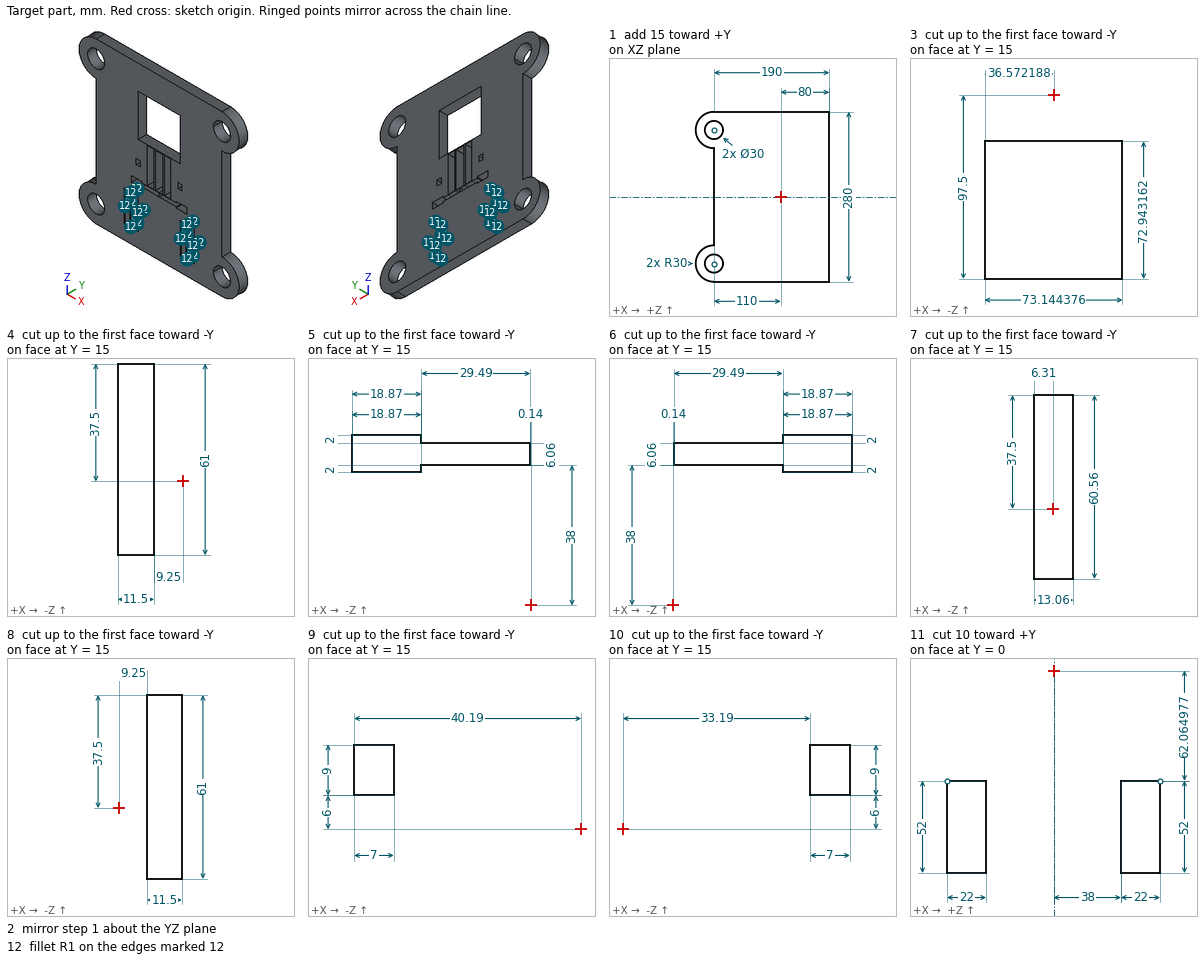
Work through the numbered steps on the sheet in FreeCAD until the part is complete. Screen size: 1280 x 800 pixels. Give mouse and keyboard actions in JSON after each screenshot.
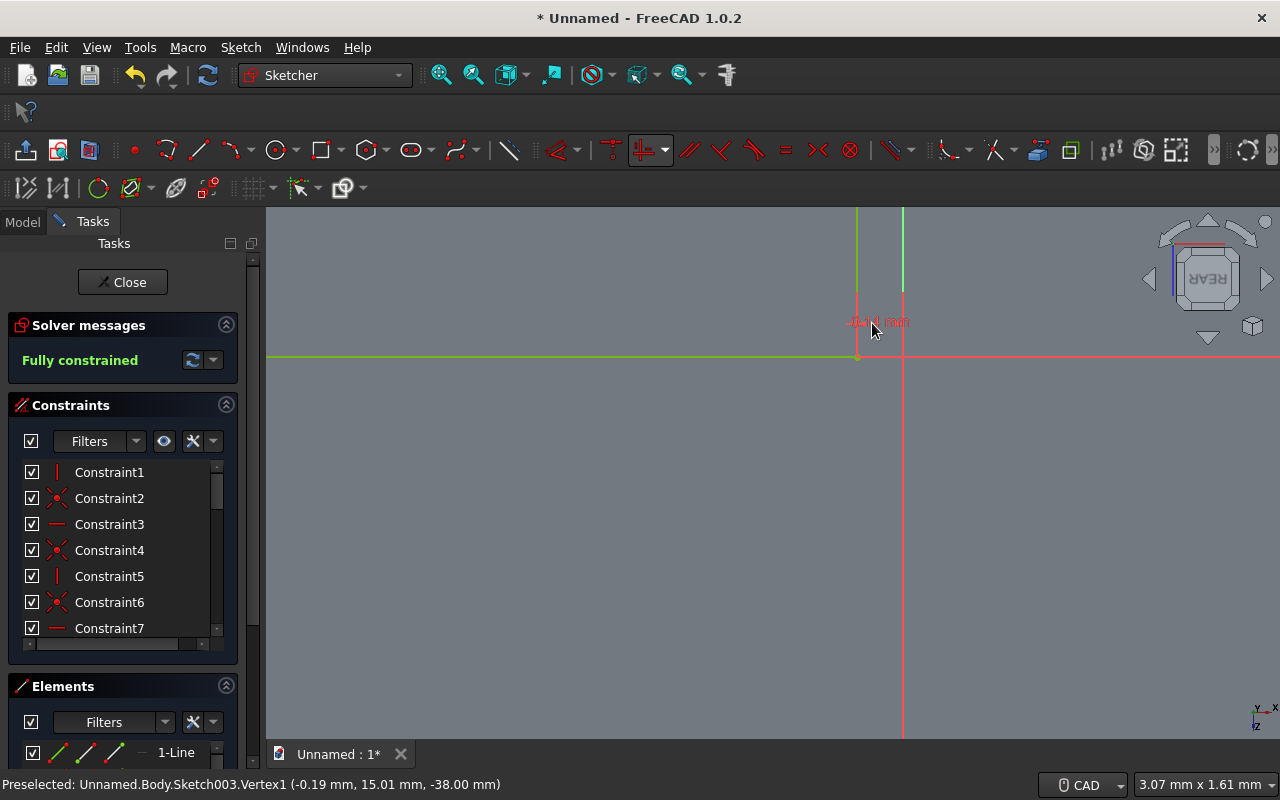
{"action": "left_click", "coordinate": [123, 282]}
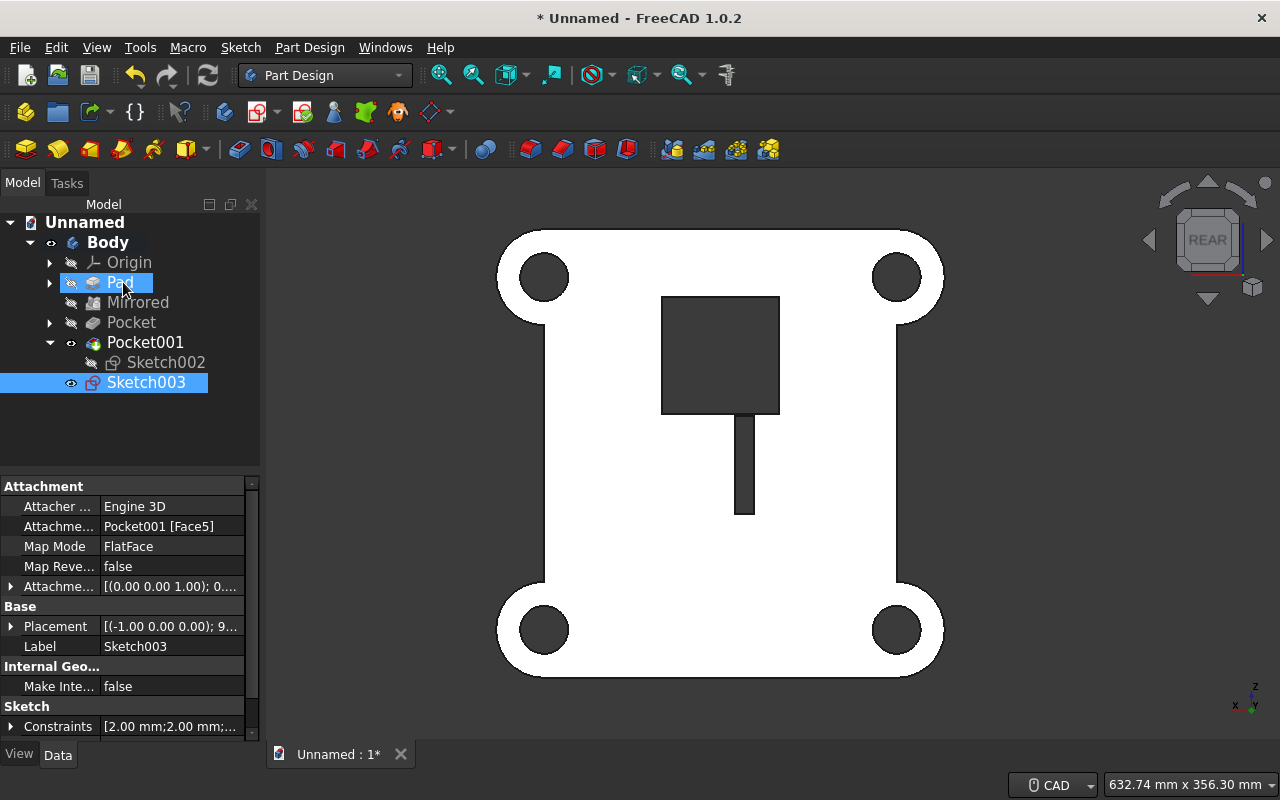
{"action": "left_click", "coordinate": [240, 150]}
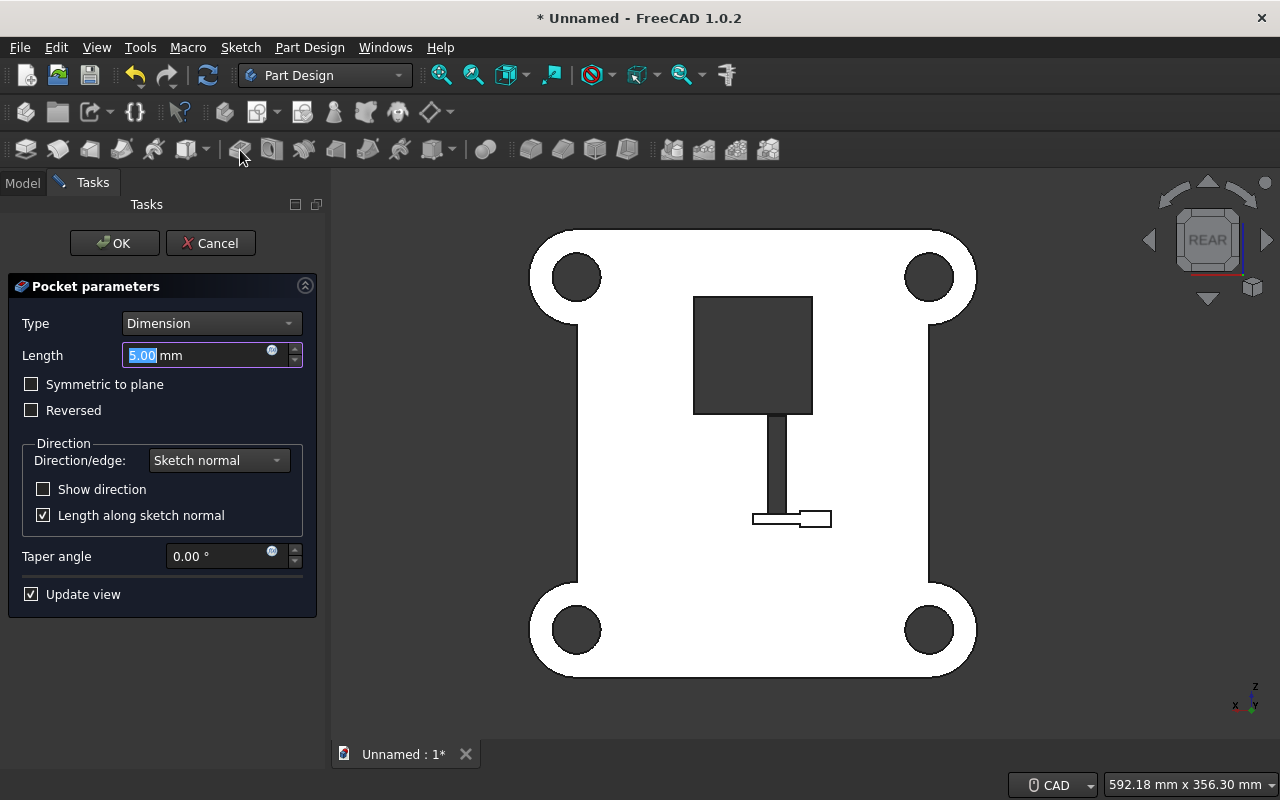
{"action": "left_click", "coordinate": [212, 324]}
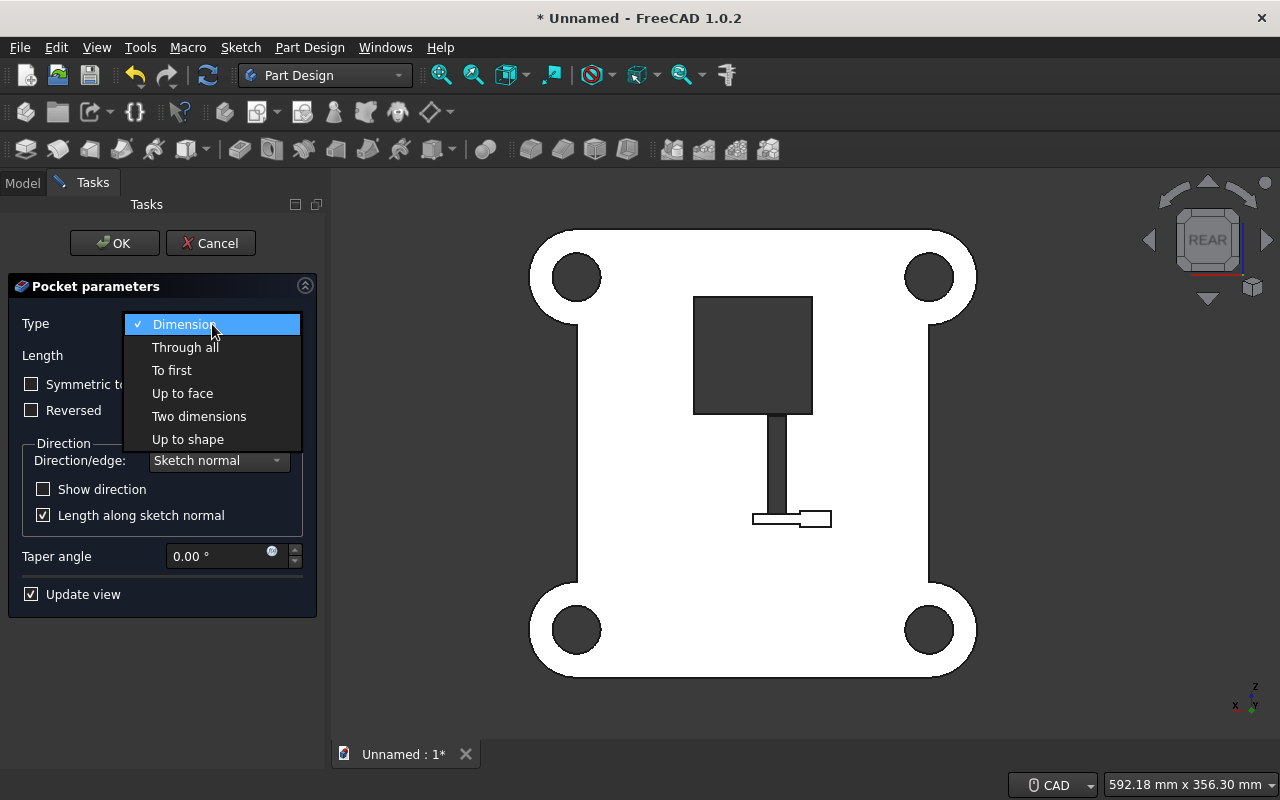
{"action": "left_click", "coordinate": [212, 370]}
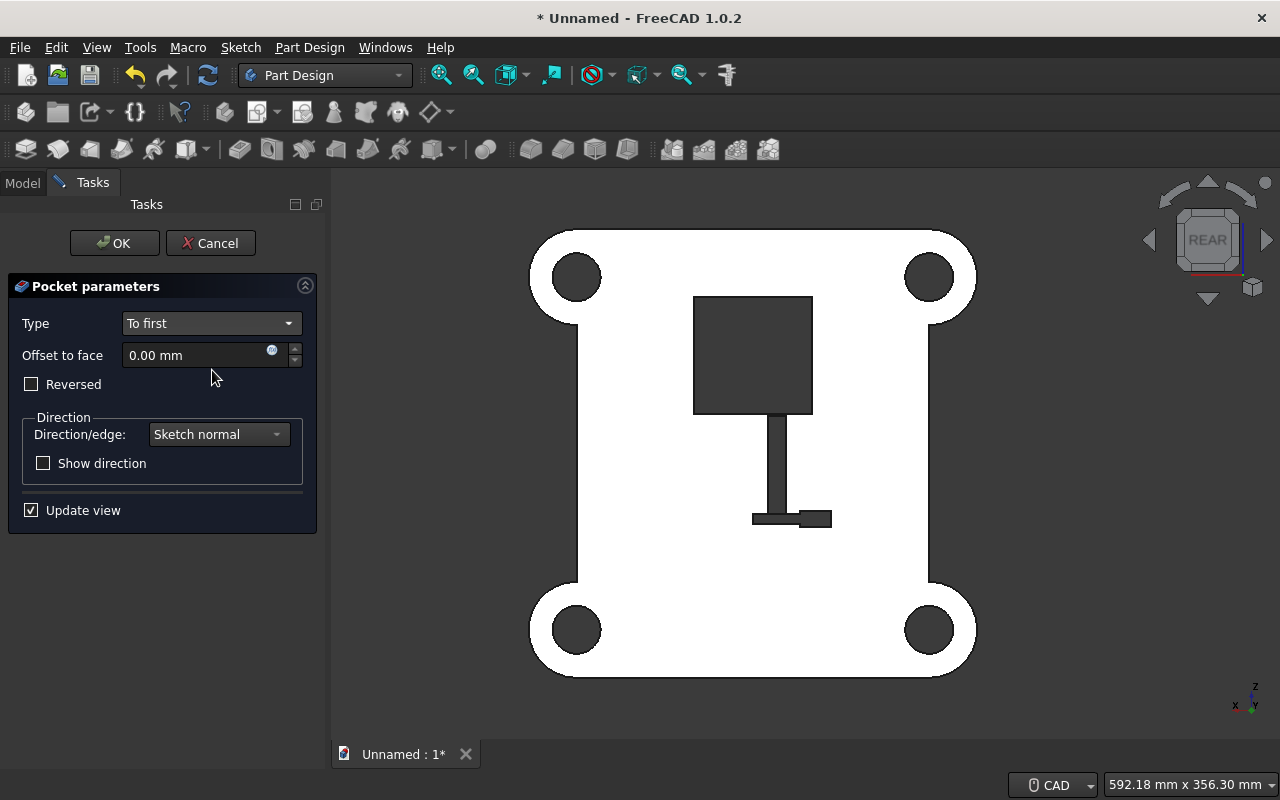
{"action": "left_click", "coordinate": [115, 243]}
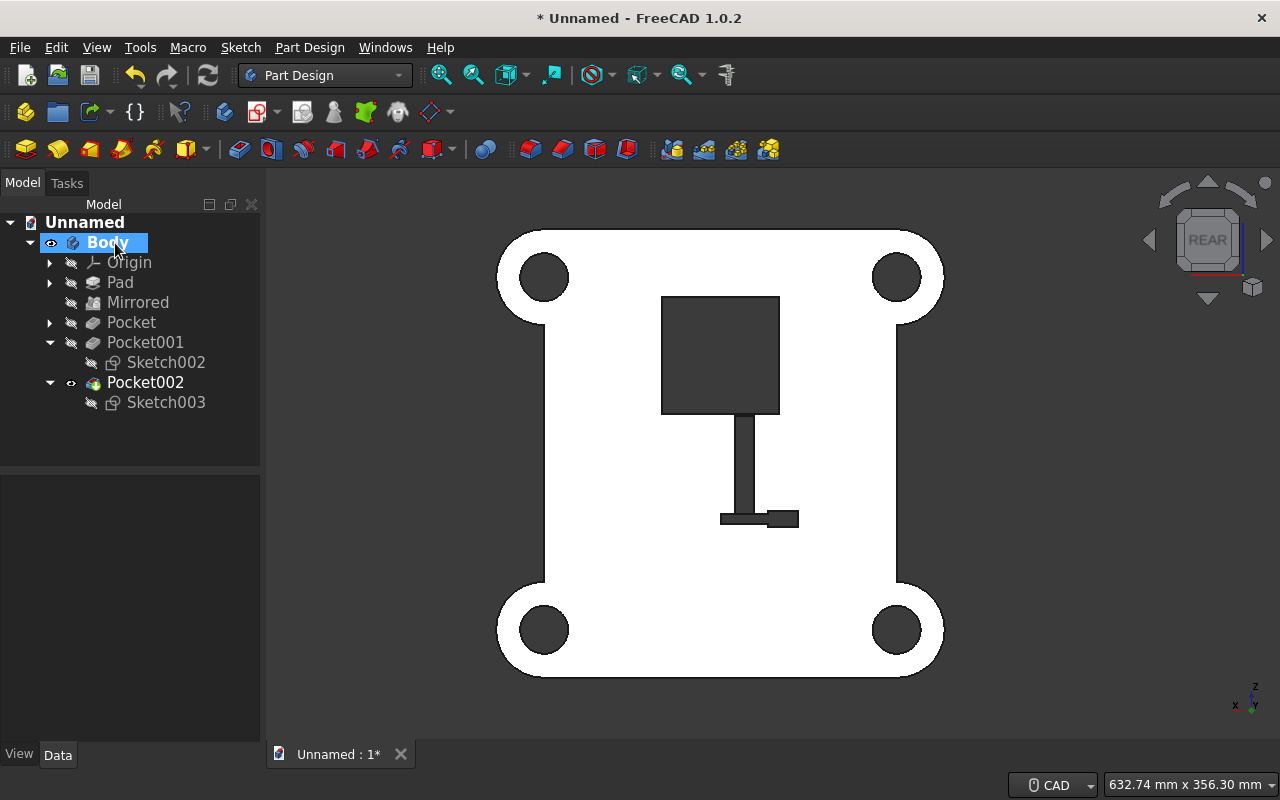
{"action": "left_click", "coordinate": [656, 581]}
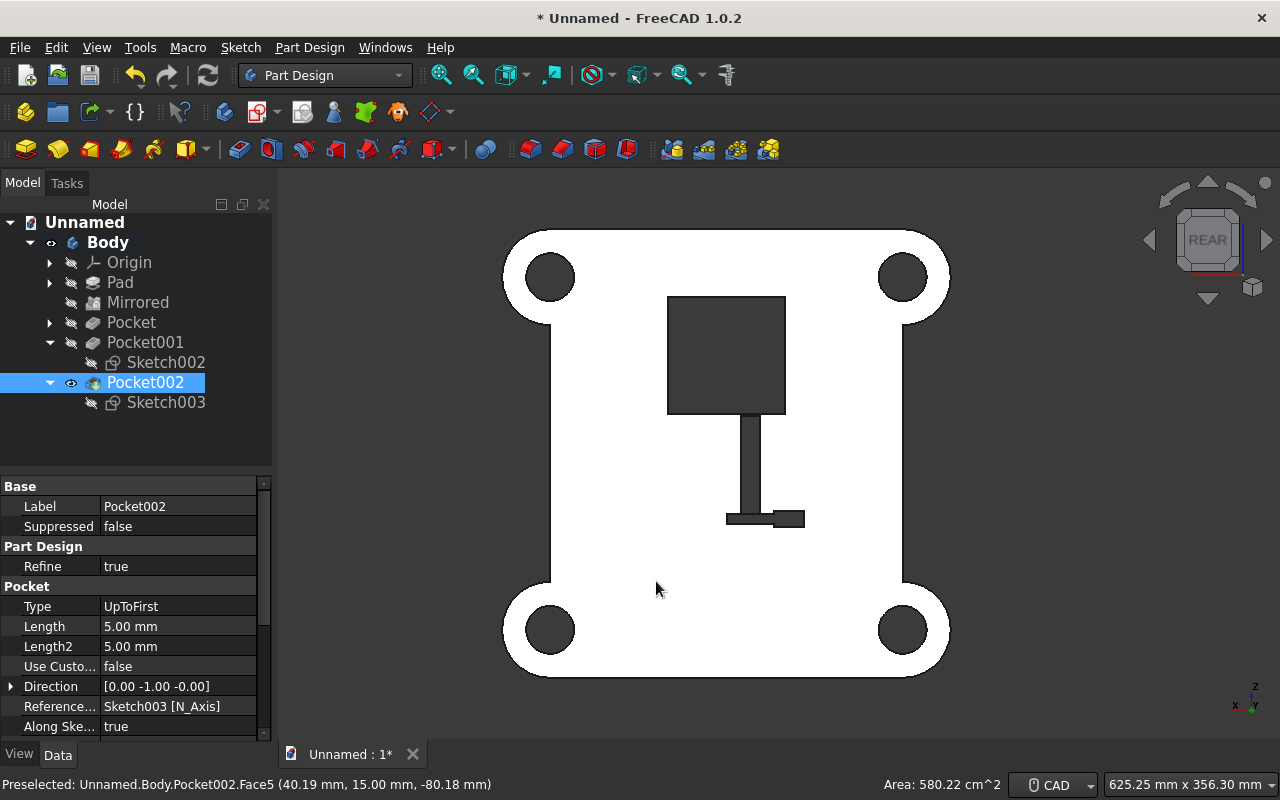
{"action": "left_click", "coordinate": [258, 112]}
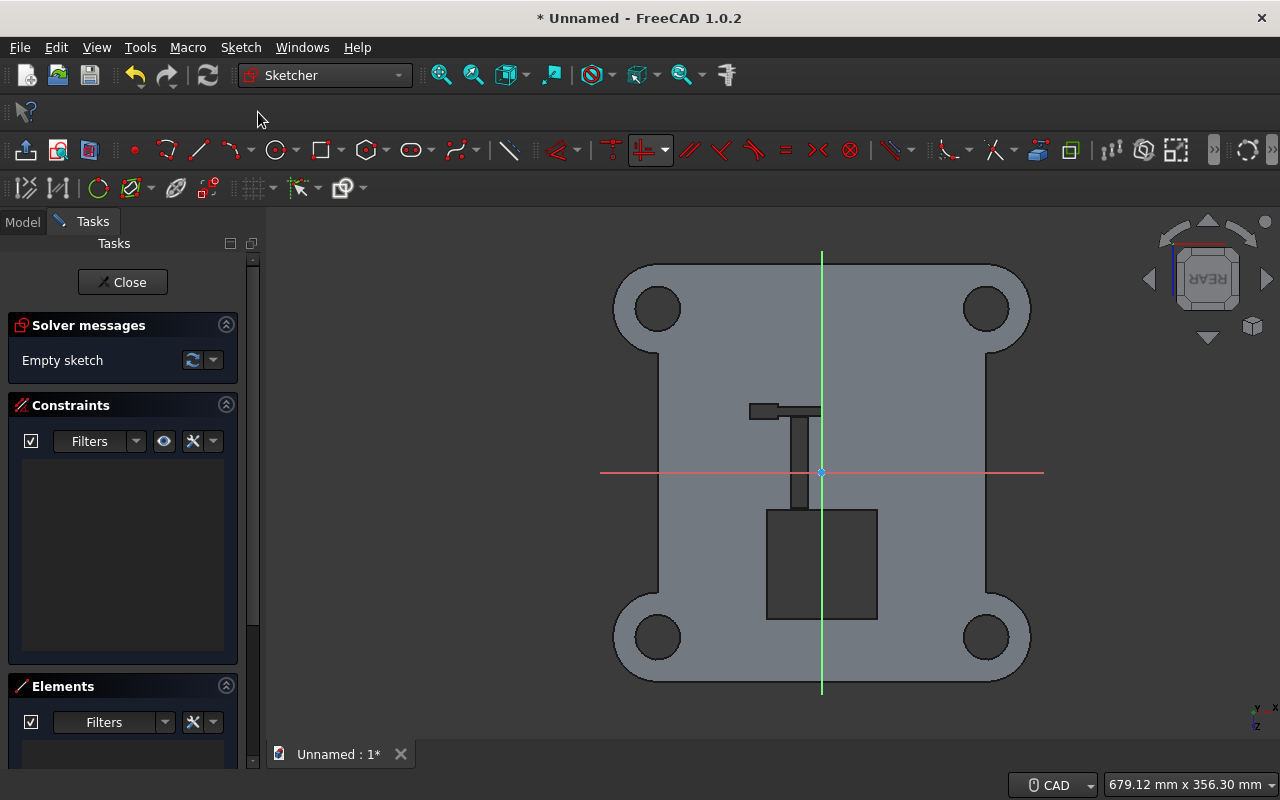
{"action": "scroll", "coordinate": [897, 430], "scroll_direction": "up", "scroll_amount": 8}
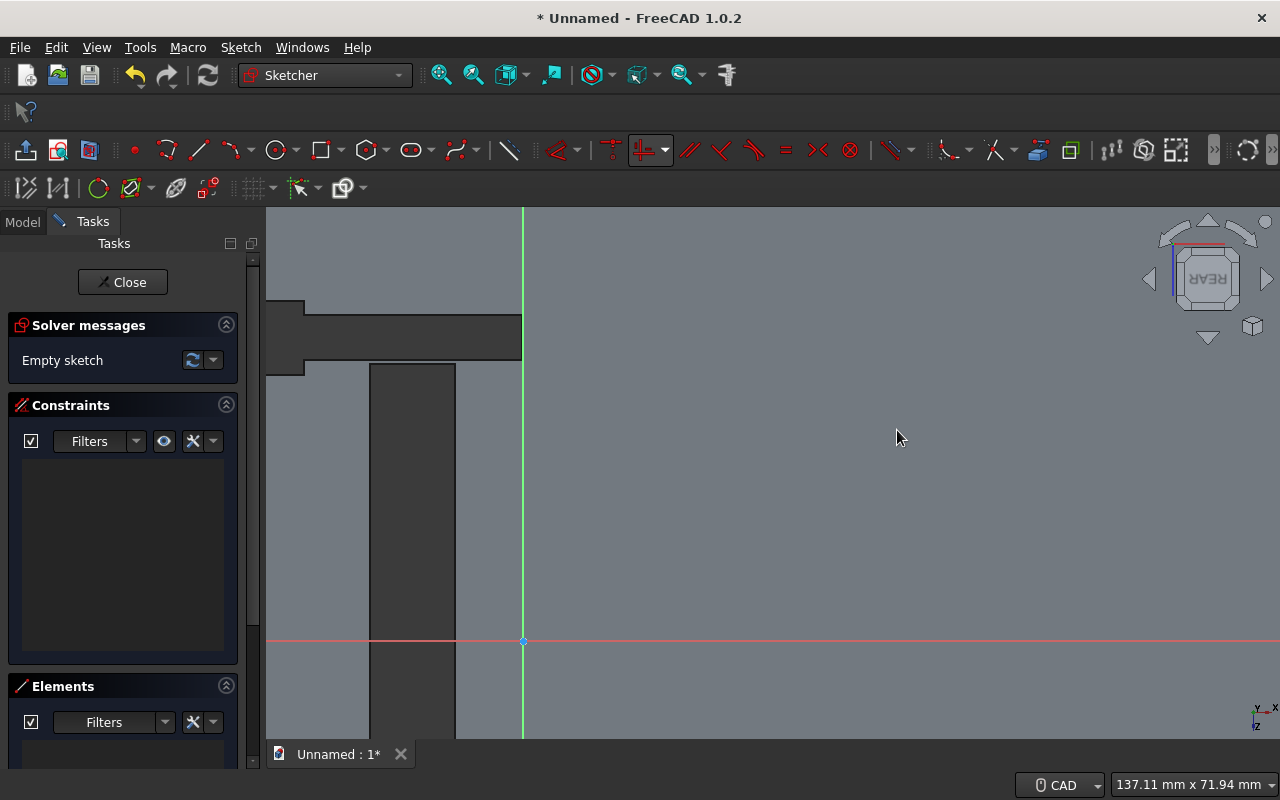
{"action": "left_click", "coordinate": [168, 150]}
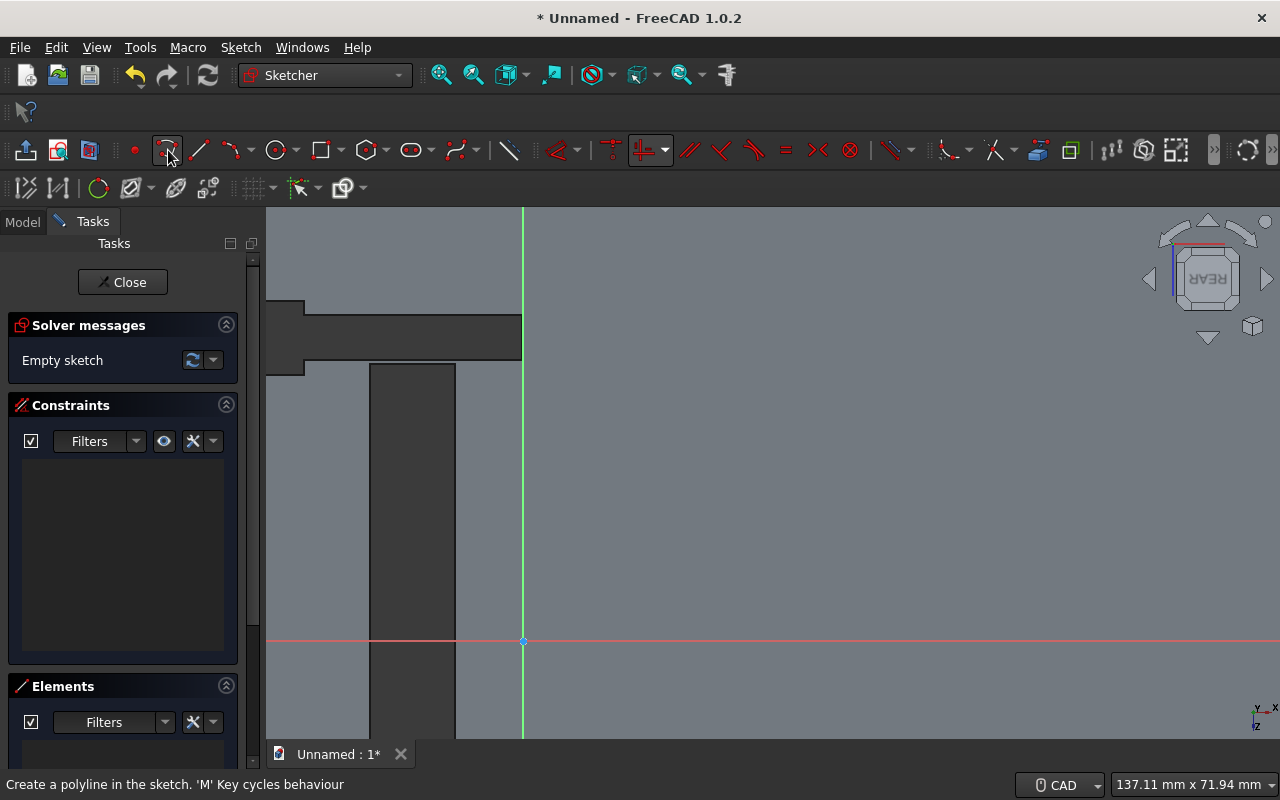
{"action": "scroll", "coordinate": [524, 360], "scroll_direction": "up", "scroll_amount": 14}